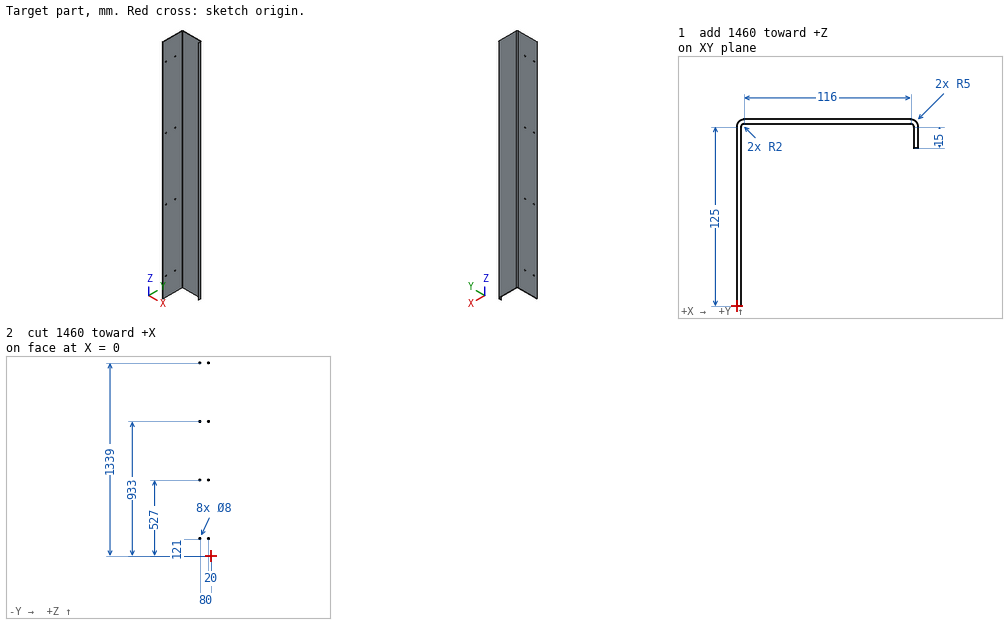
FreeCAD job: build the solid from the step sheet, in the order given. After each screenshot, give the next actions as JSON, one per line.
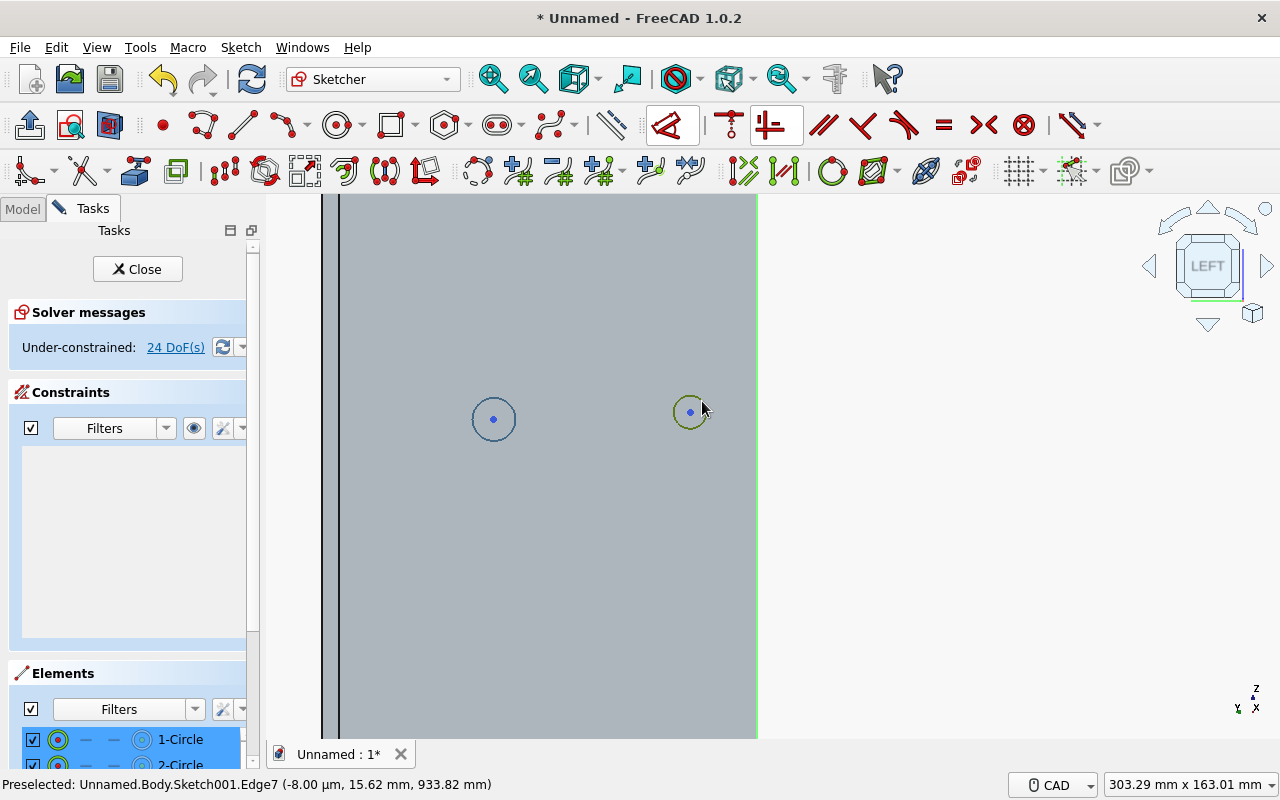
{"action": "scroll", "coordinate": [712, 401], "scroll_direction": "down", "scroll_amount": 13}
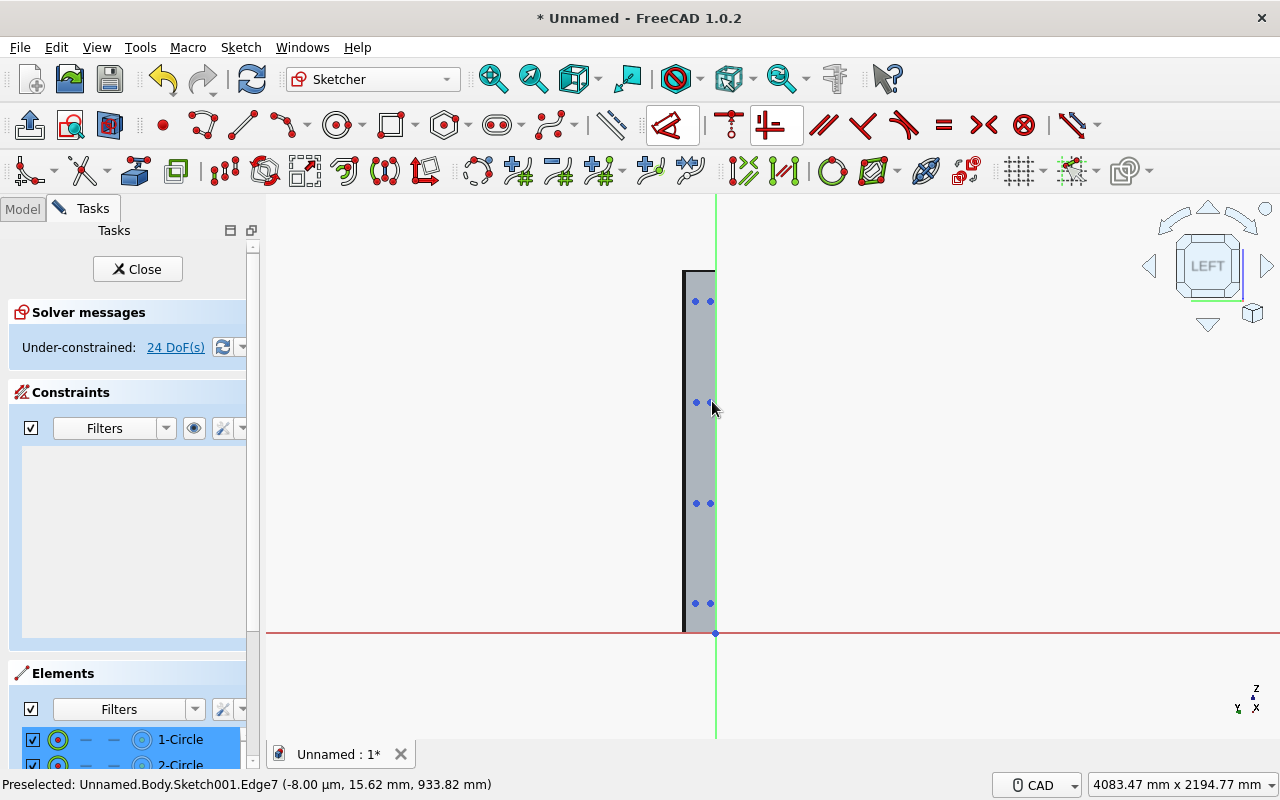
{"action": "scroll", "coordinate": [712, 502], "scroll_direction": "up", "scroll_amount": 12}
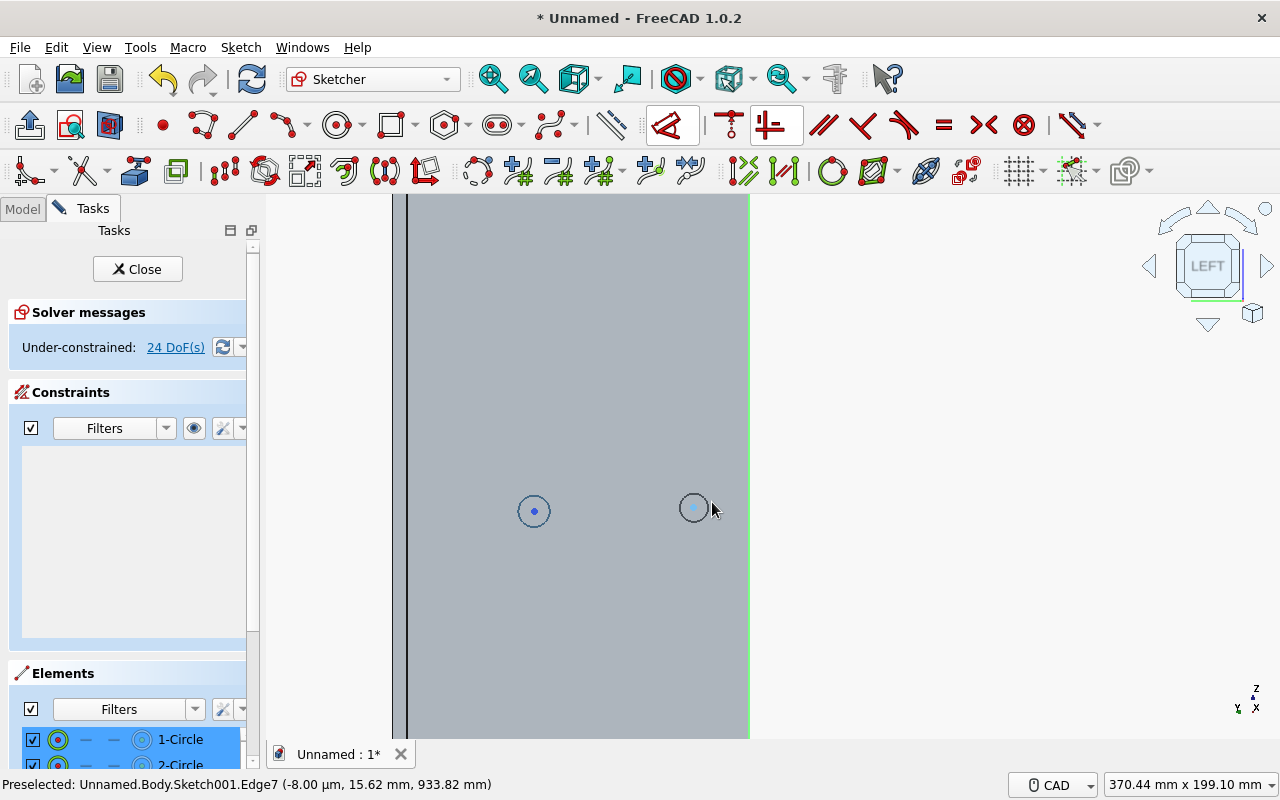
{"action": "left_click", "coordinate": [704, 498]}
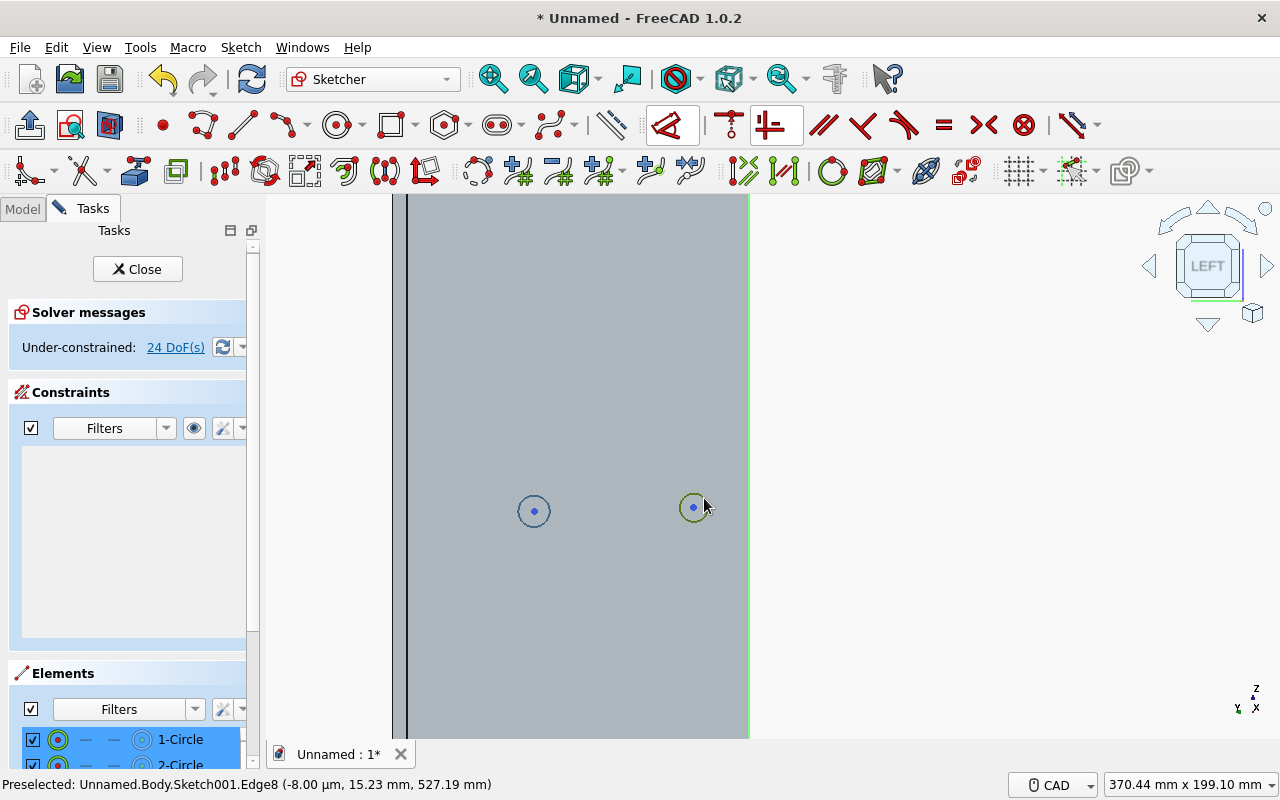
{"action": "key", "text": "e"}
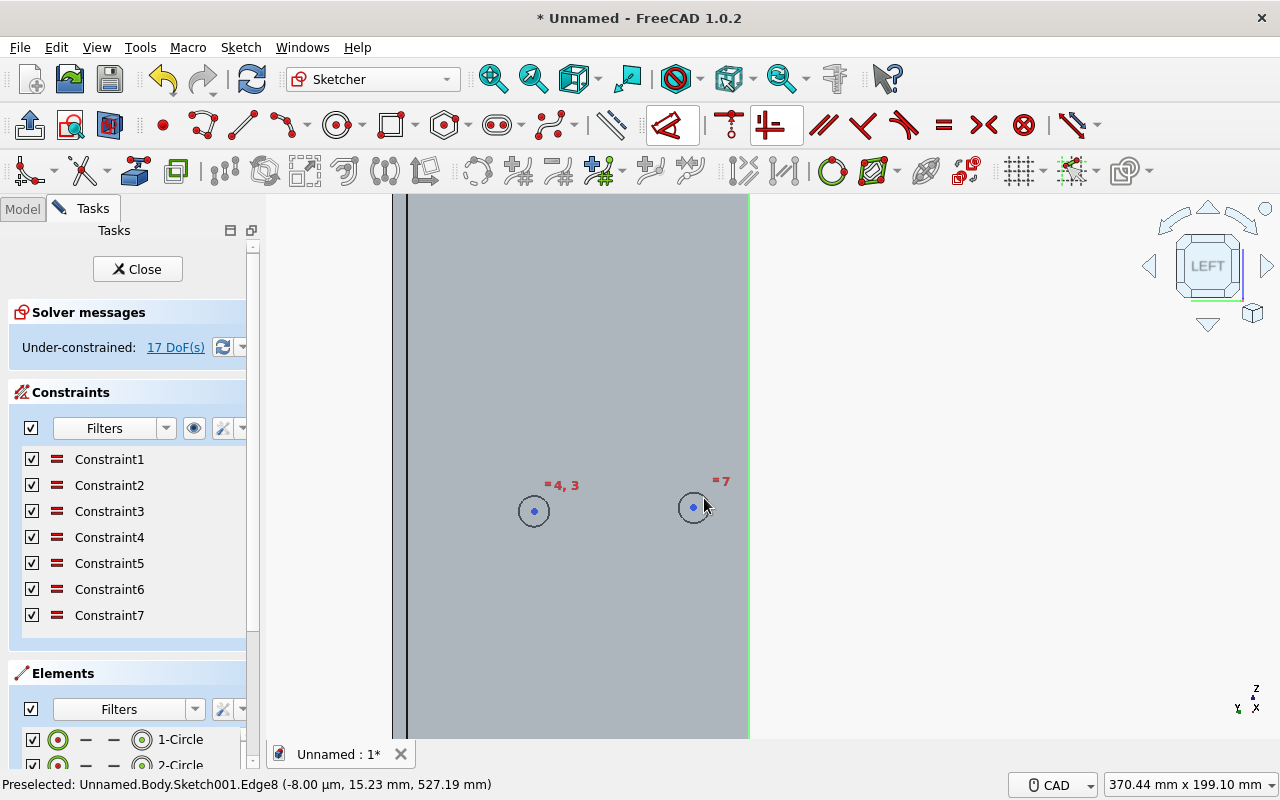
{"action": "scroll", "coordinate": [712, 502], "scroll_direction": "down", "scroll_amount": 12}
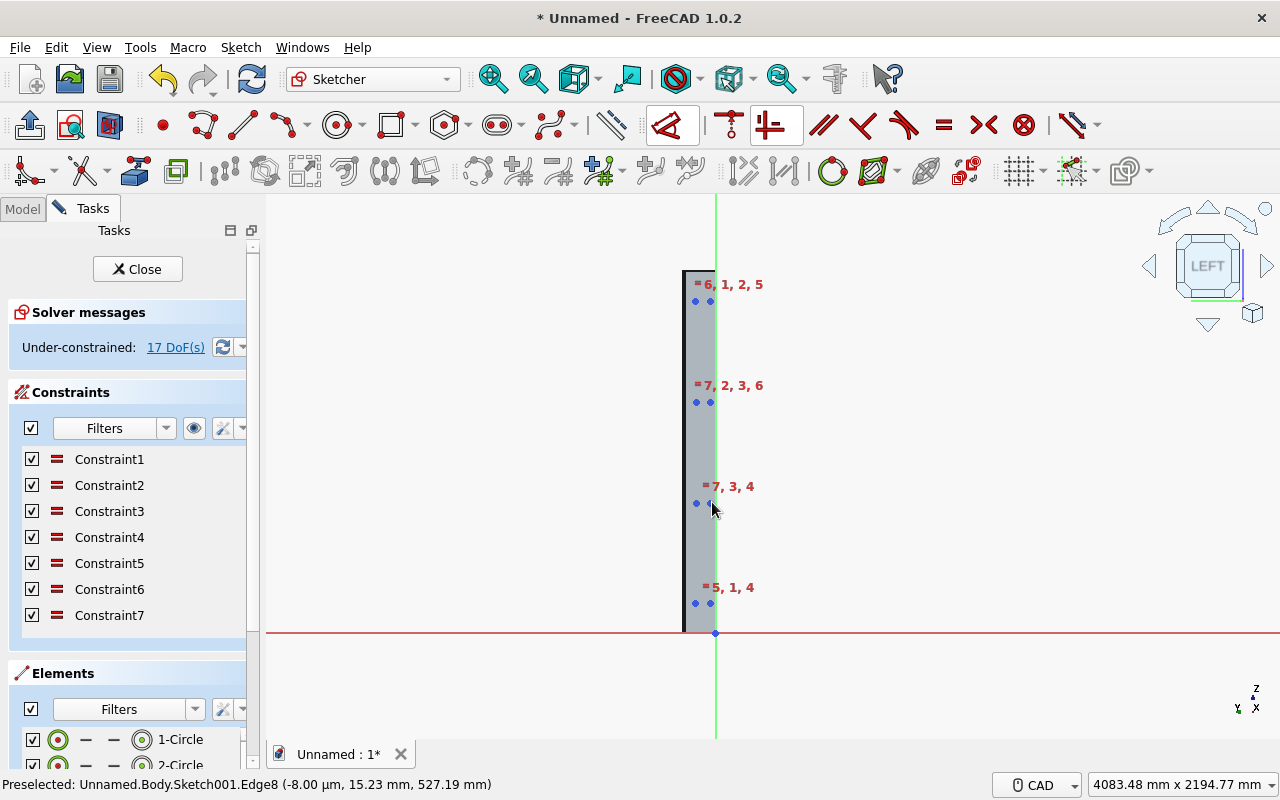
{"action": "left_click", "coordinate": [696, 604]}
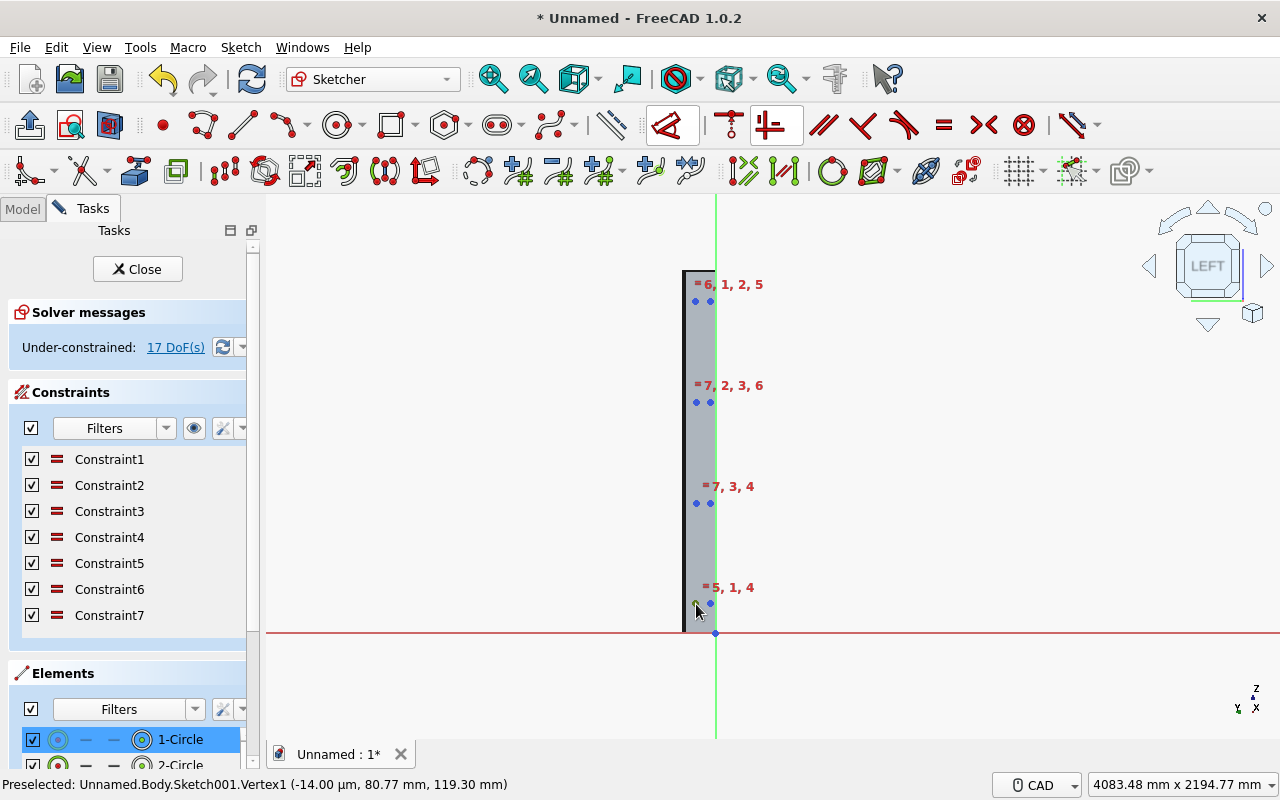
{"action": "left_click", "coordinate": [696, 302]}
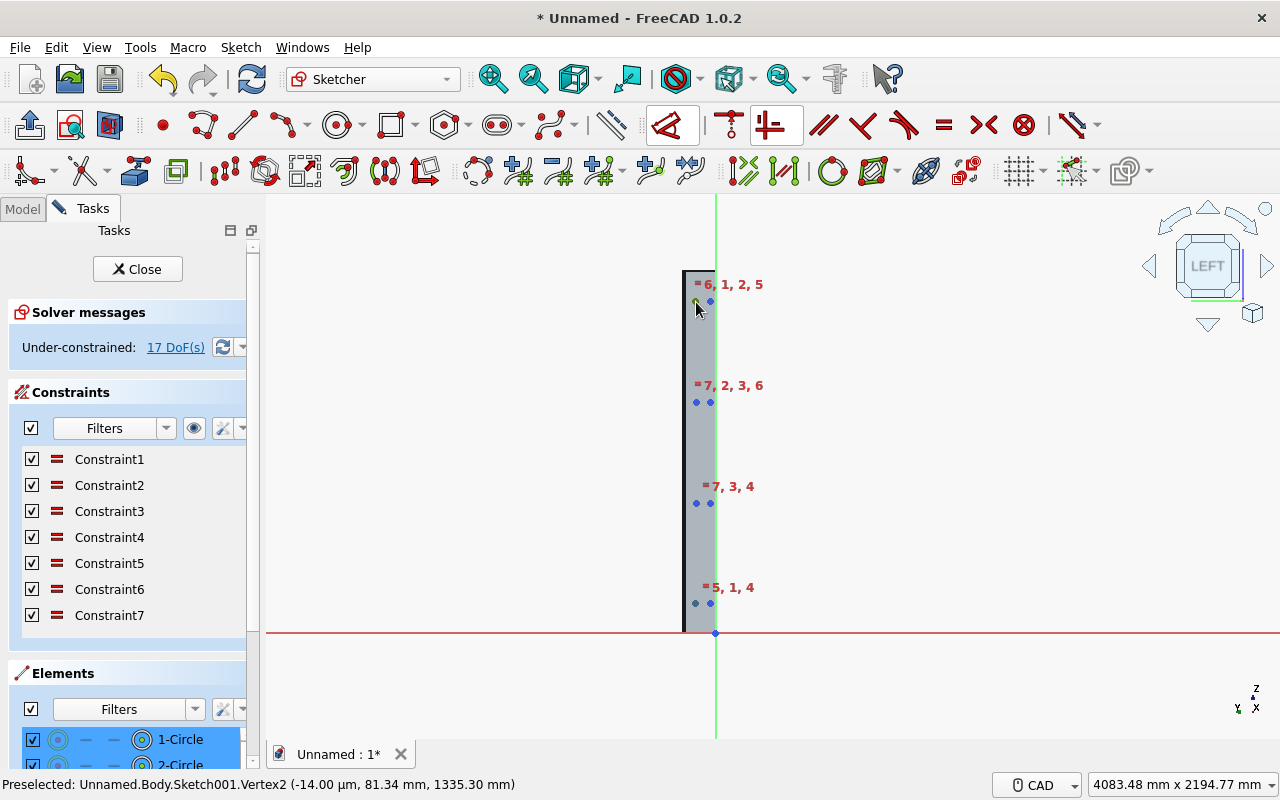
{"action": "key", "text": "v"}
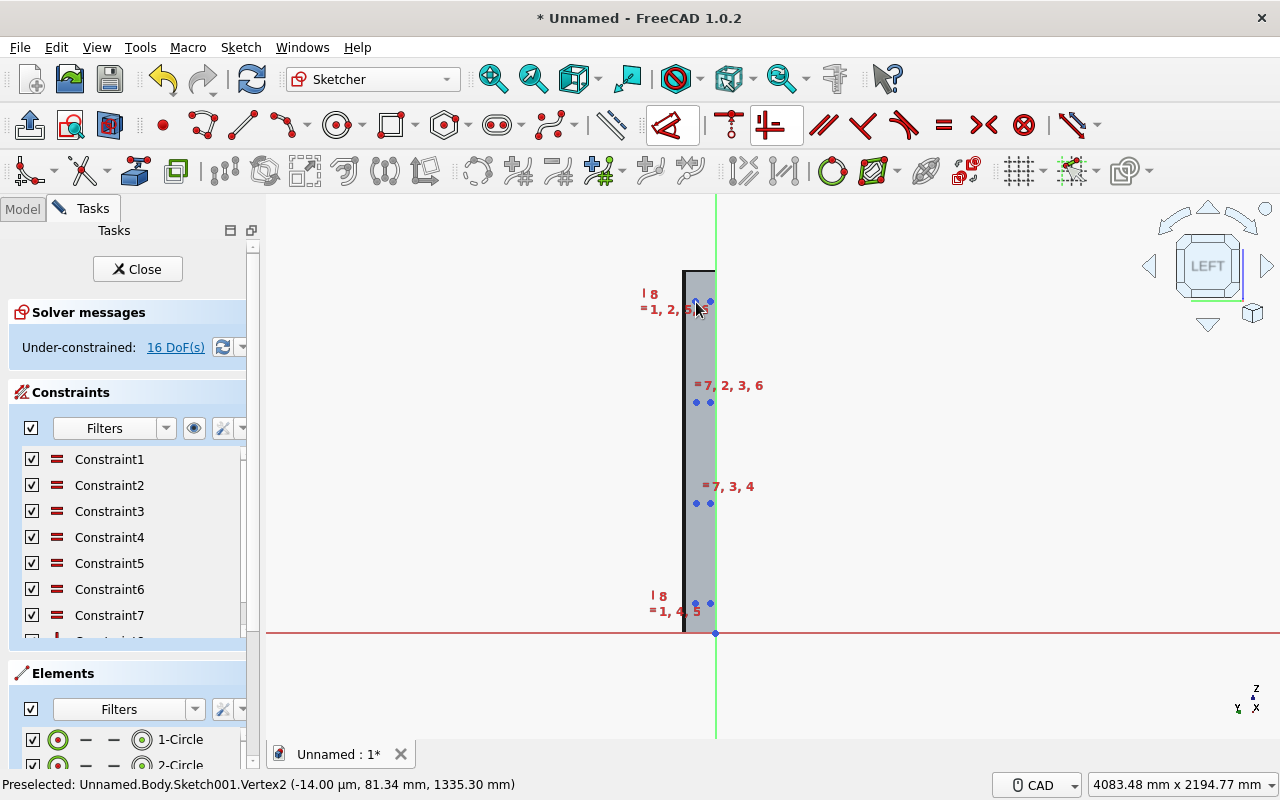
{"action": "scroll", "coordinate": [696, 302], "scroll_direction": "up", "scroll_amount": 4}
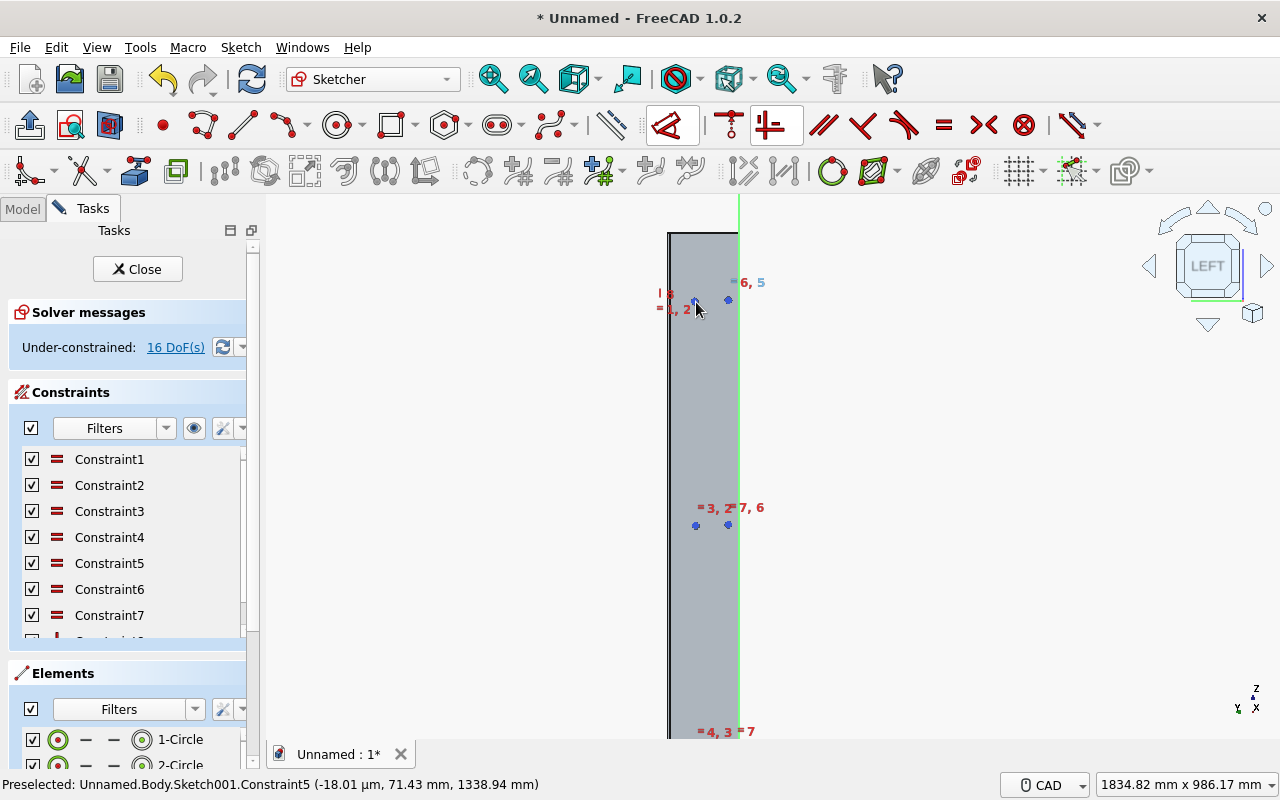
{"action": "left_click", "coordinate": [695, 302]}